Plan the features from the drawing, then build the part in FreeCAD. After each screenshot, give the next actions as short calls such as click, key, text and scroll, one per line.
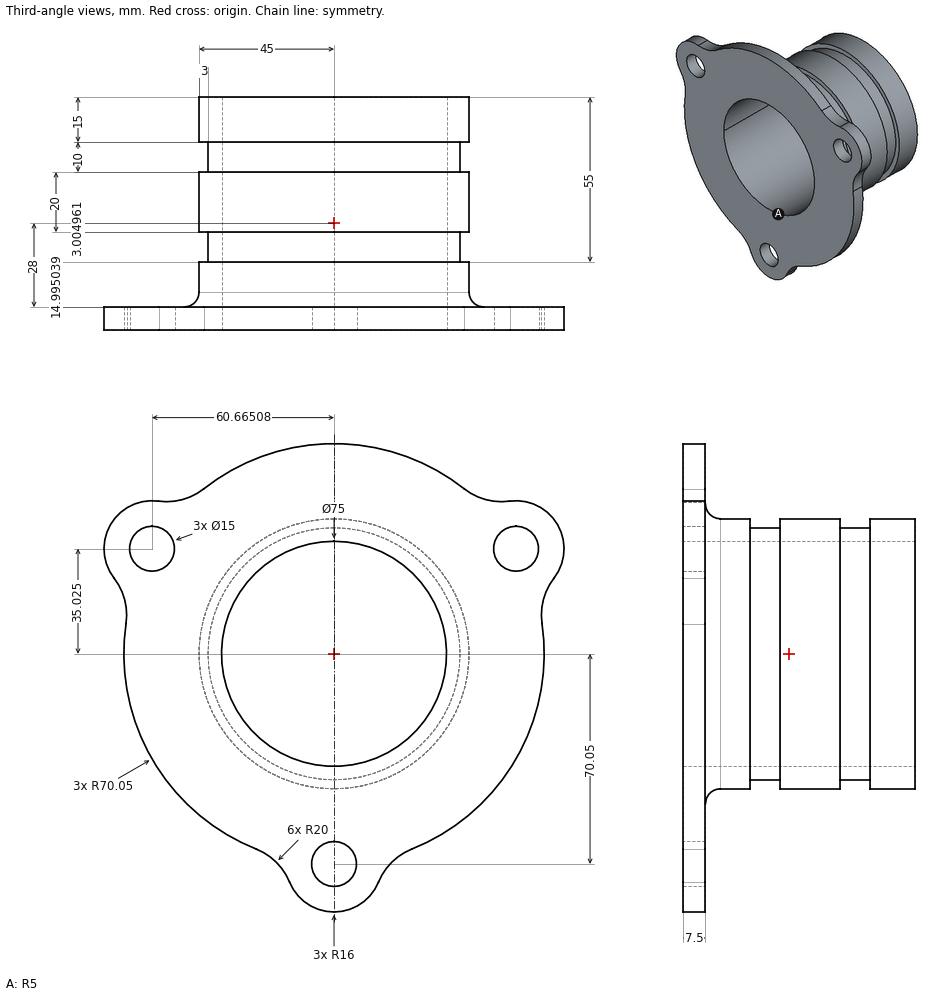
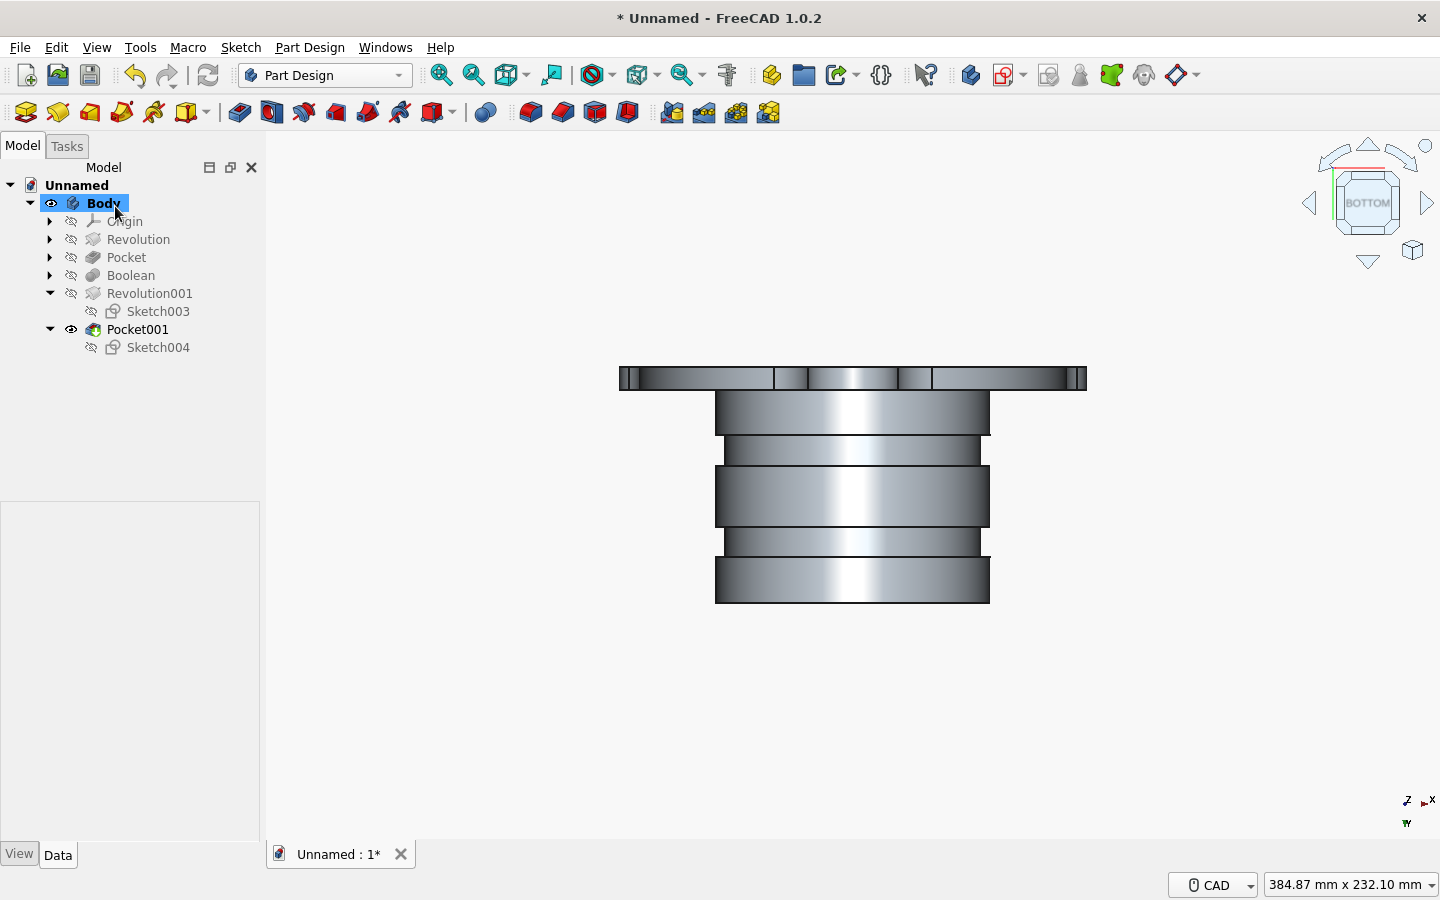
key(4)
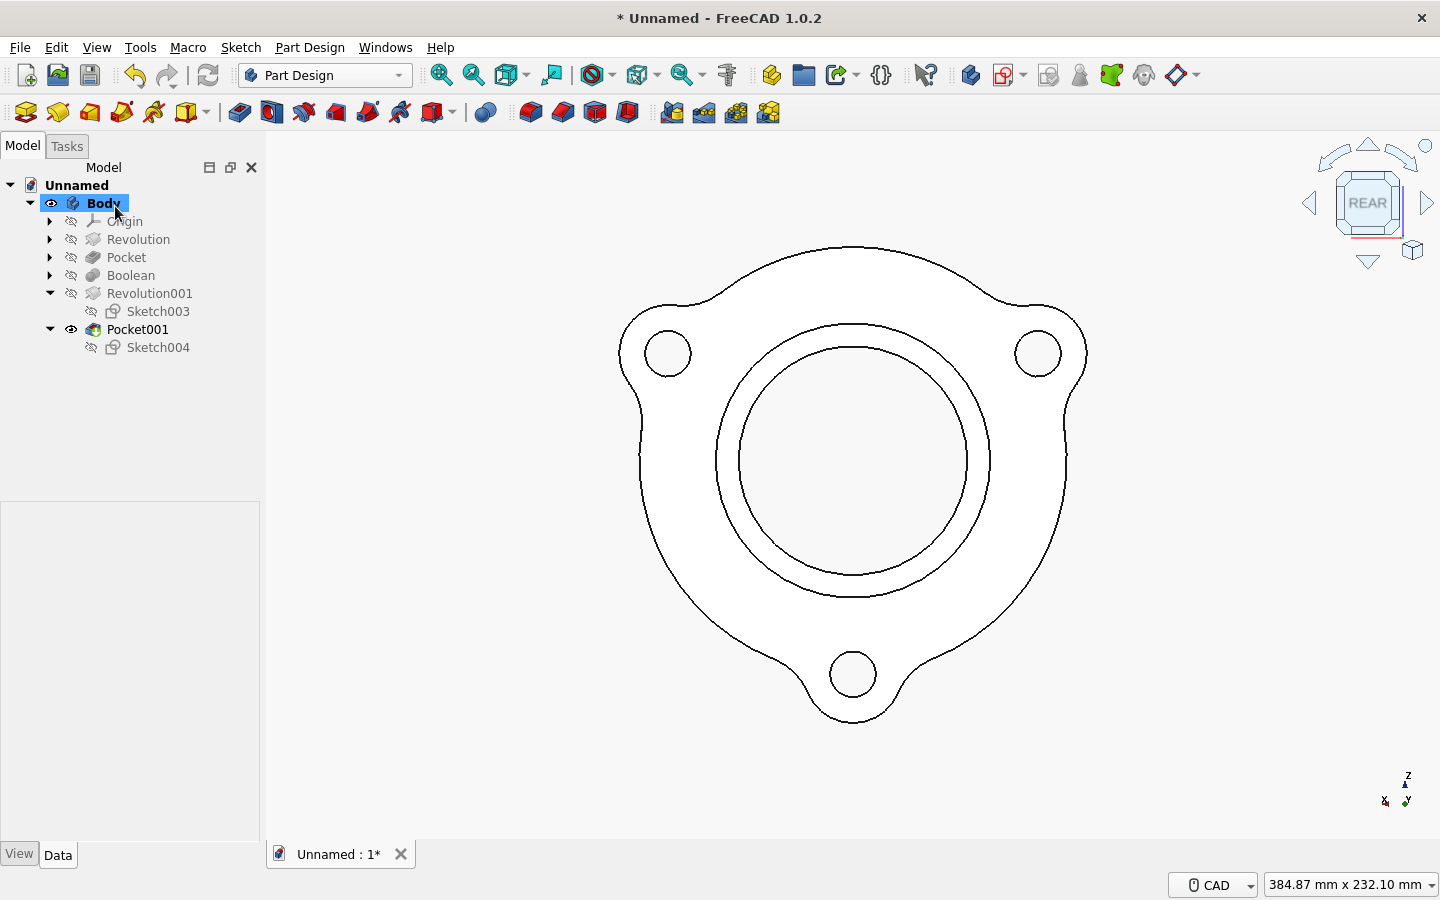
key(6)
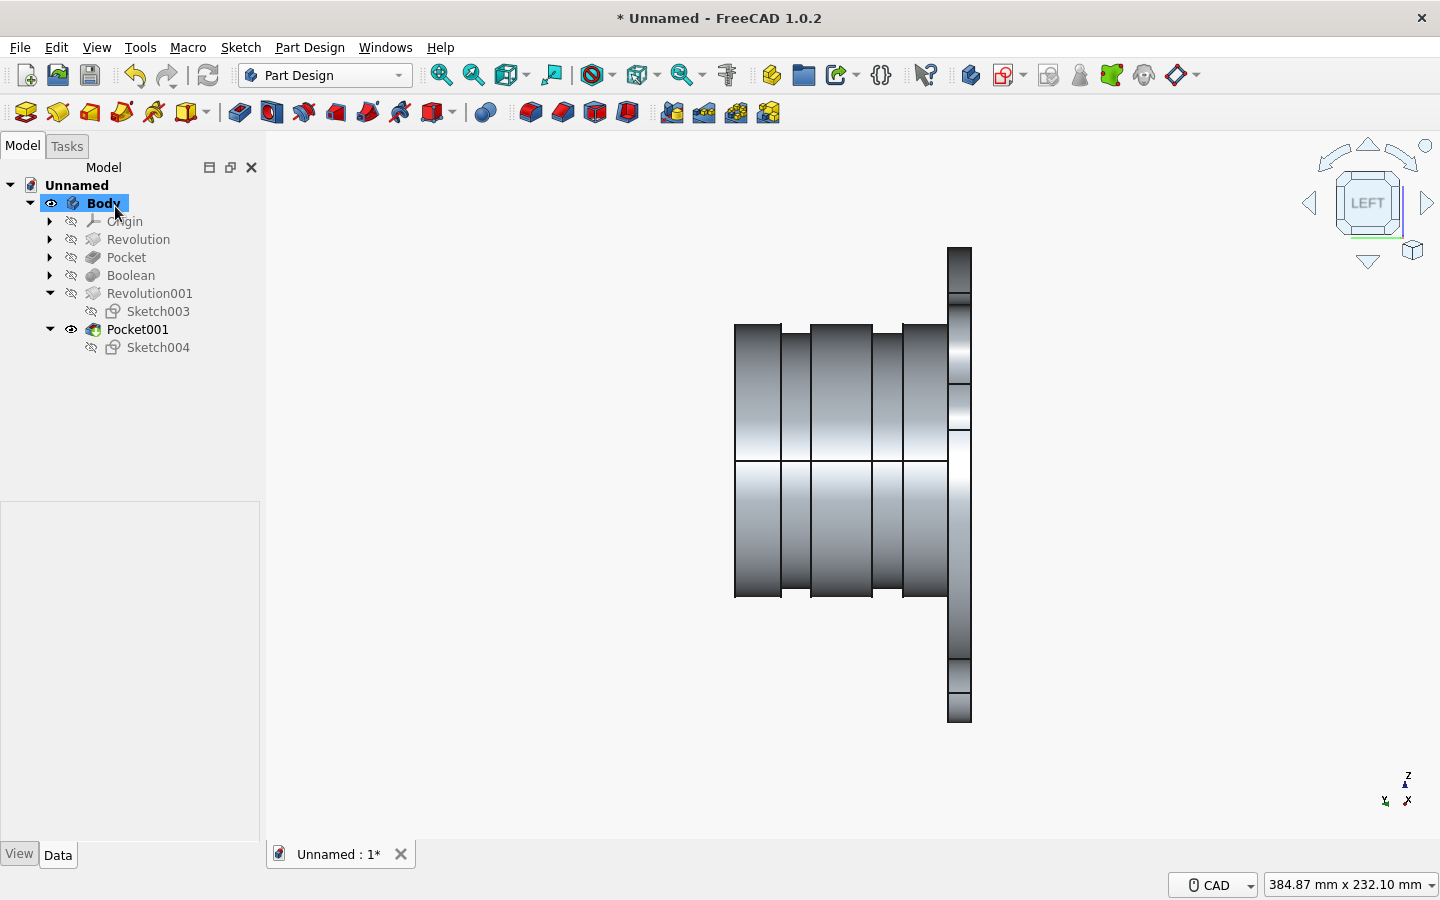
key(v)
key(3)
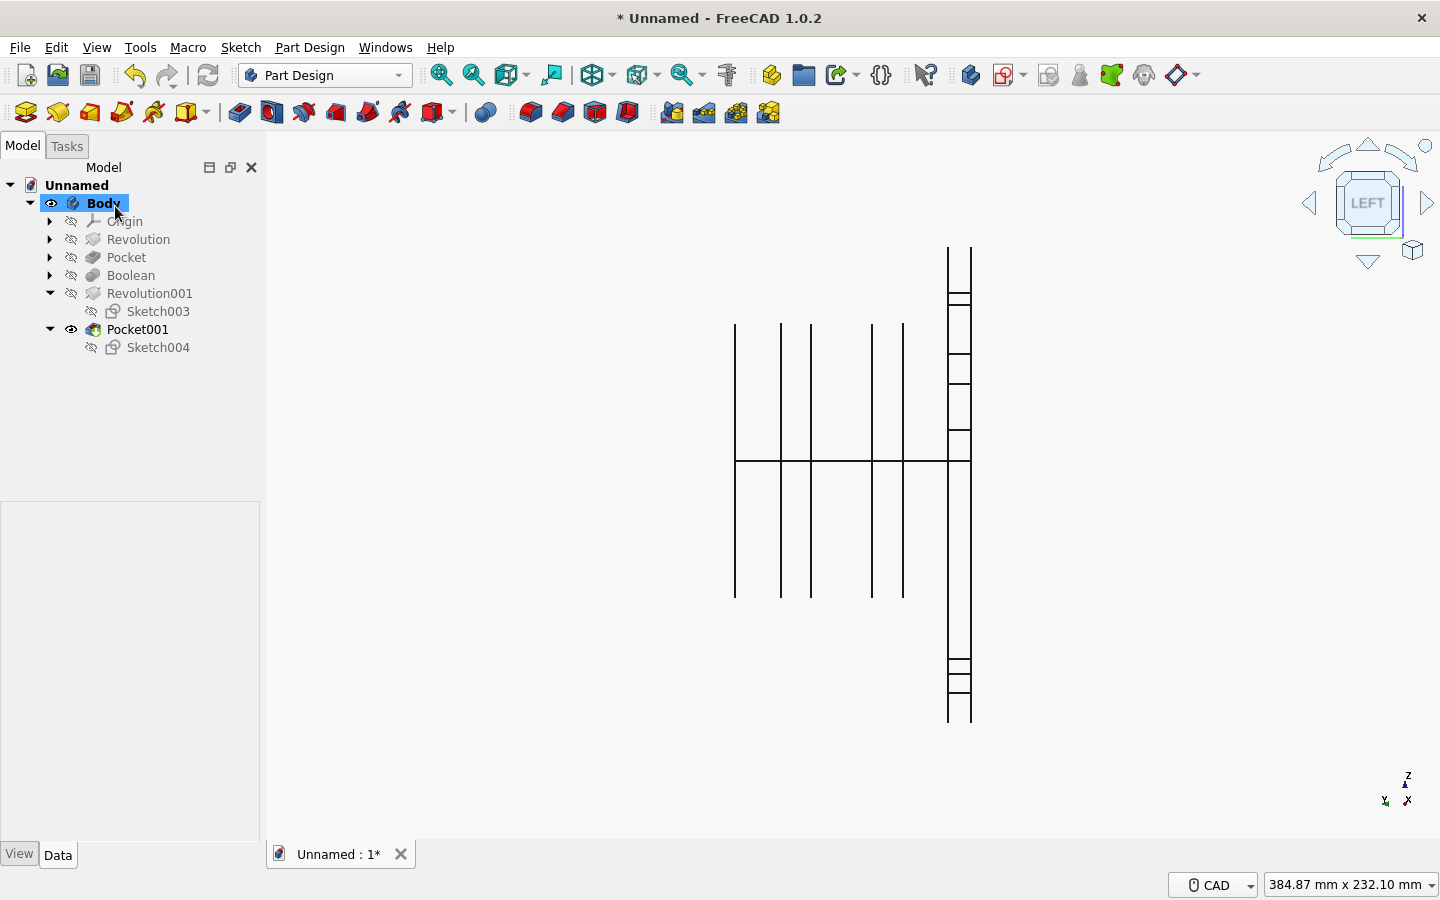
key(0)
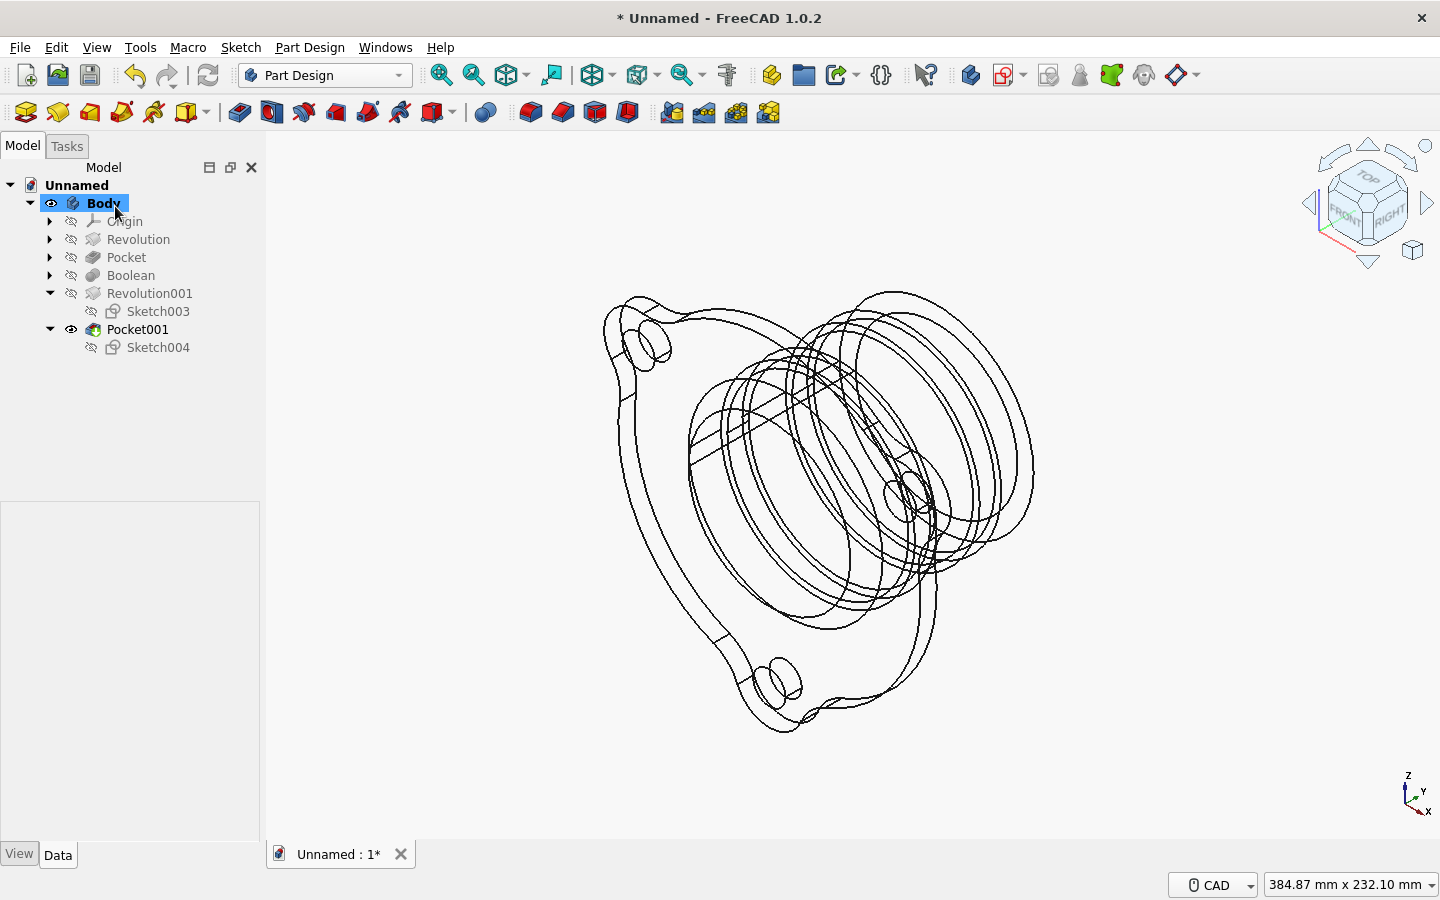
click(883, 559)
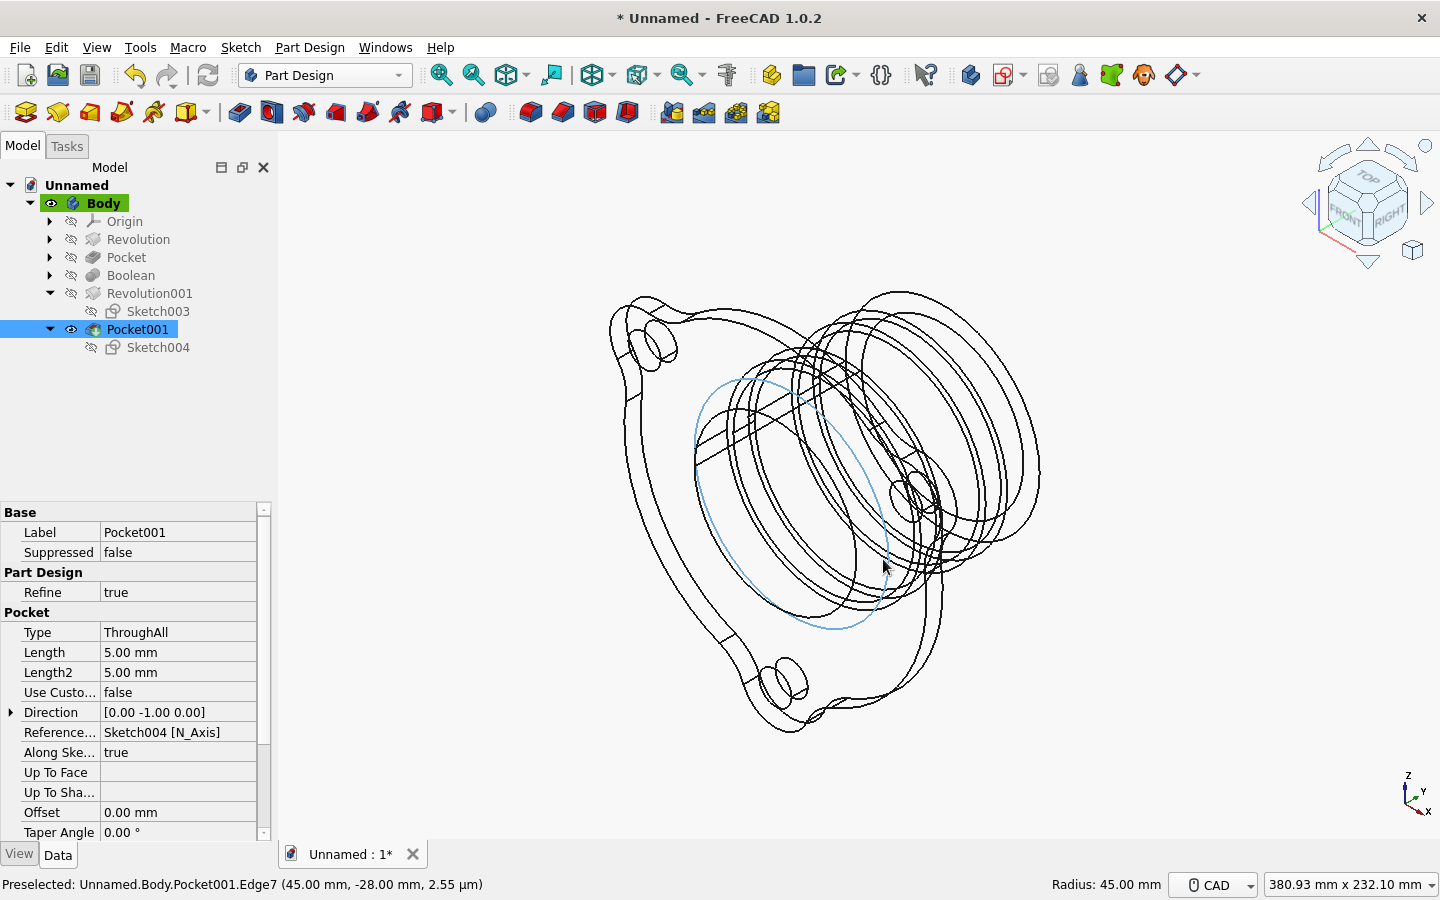
key(v)
key(1)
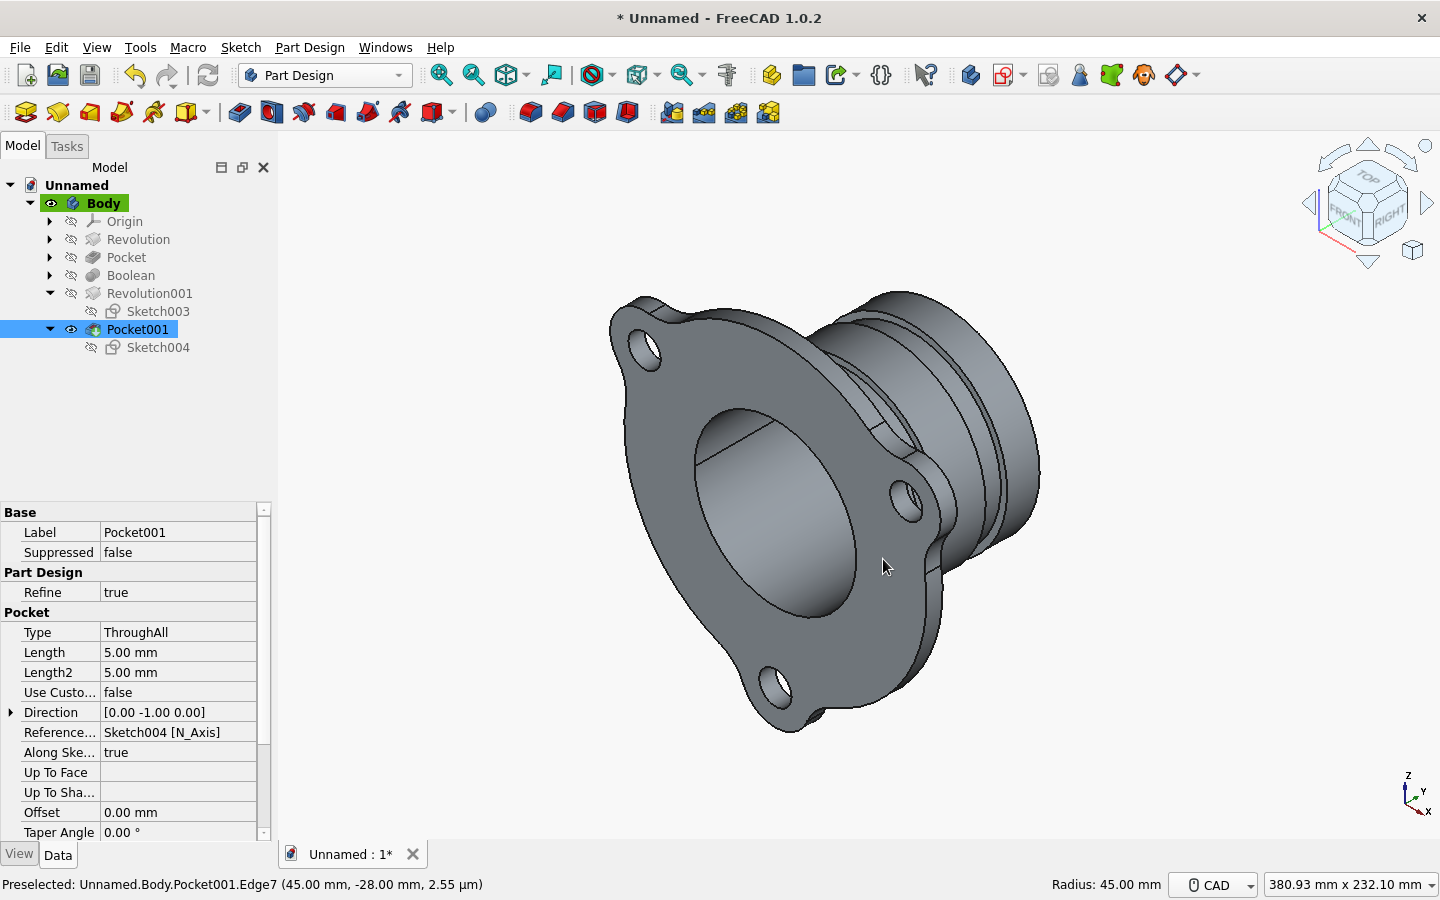
click(532, 112)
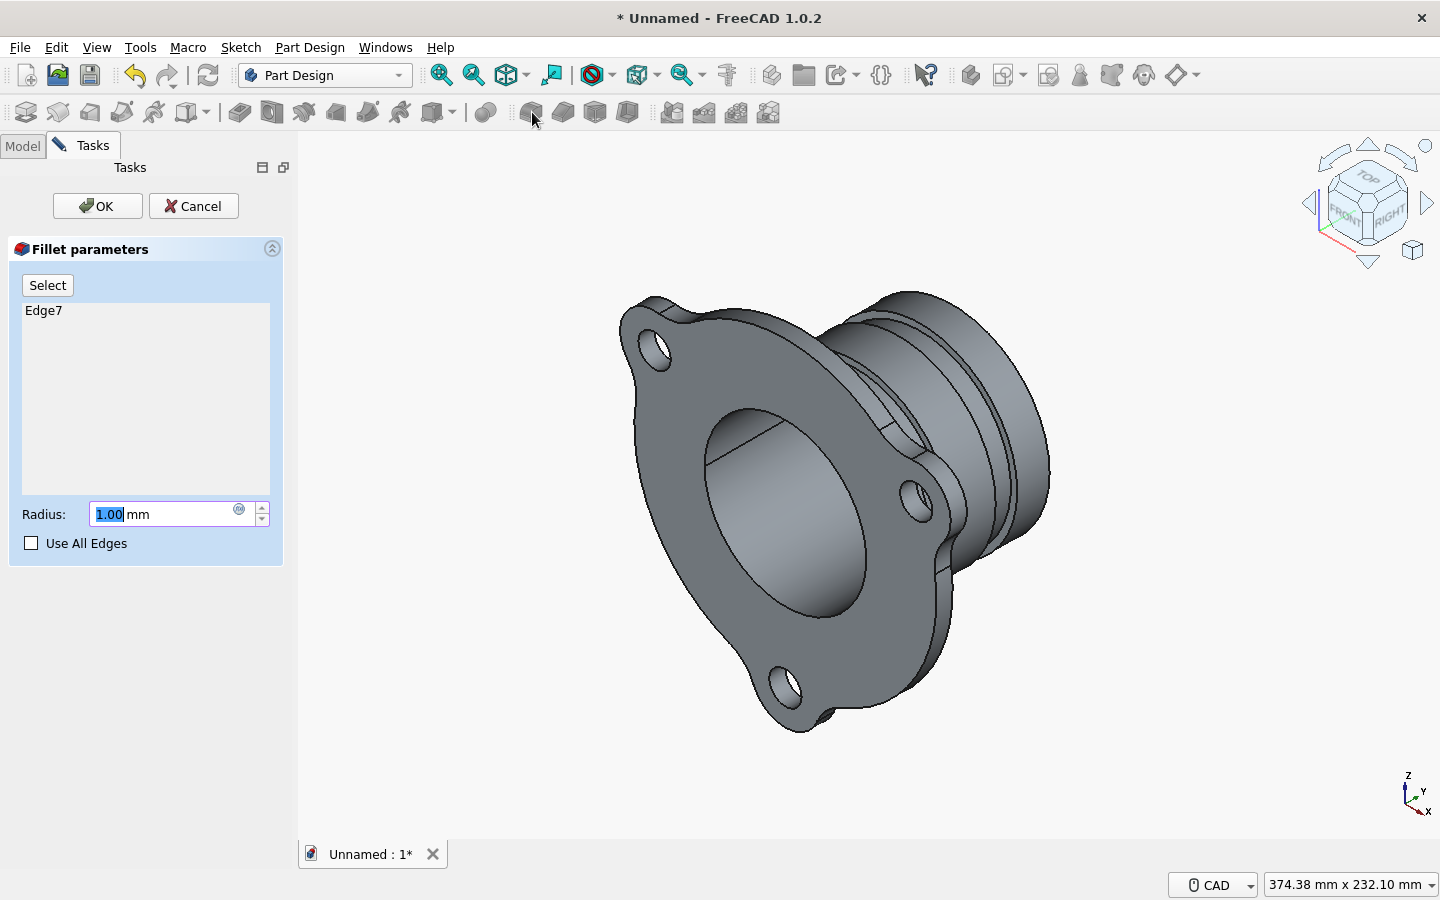
text(5)
key(Tab)